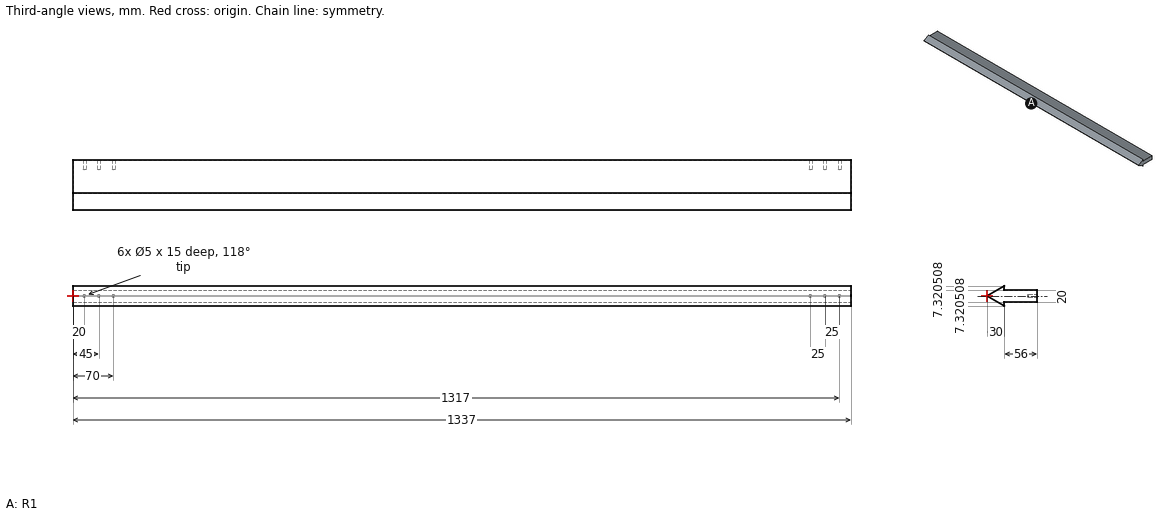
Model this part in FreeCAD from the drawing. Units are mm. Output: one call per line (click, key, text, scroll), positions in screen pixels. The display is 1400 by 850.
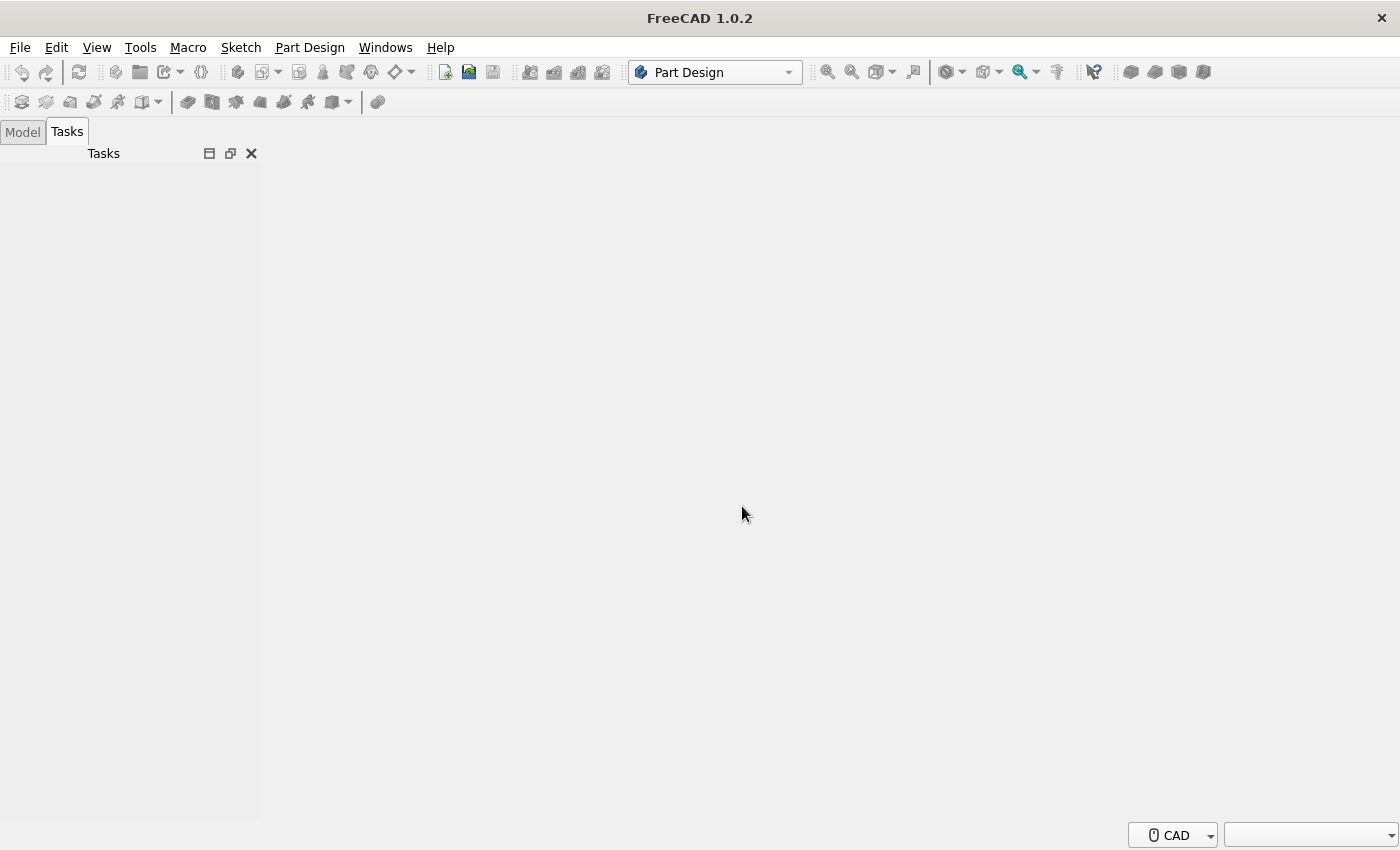
click(446, 72)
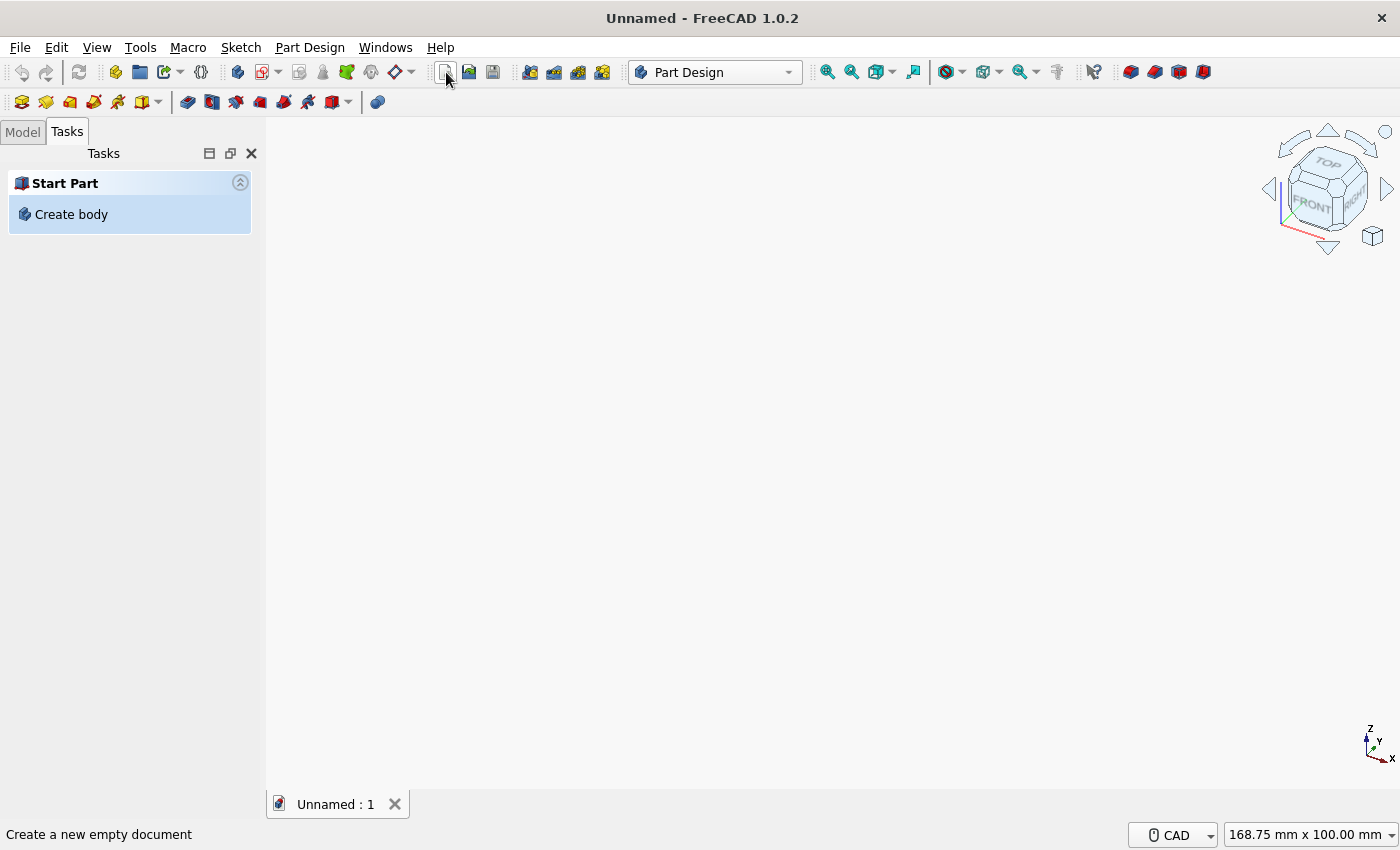
click(262, 72)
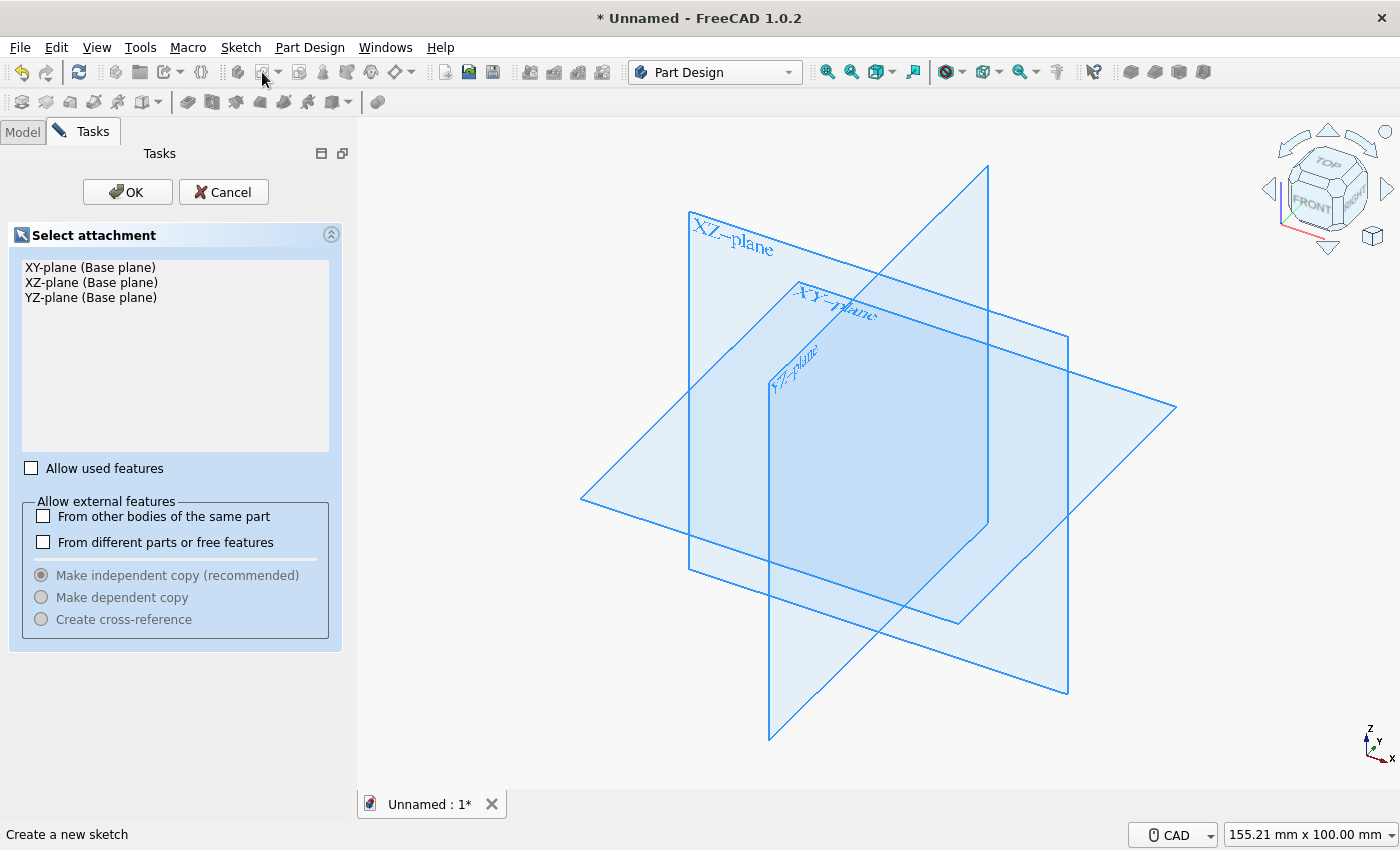
click(82, 298)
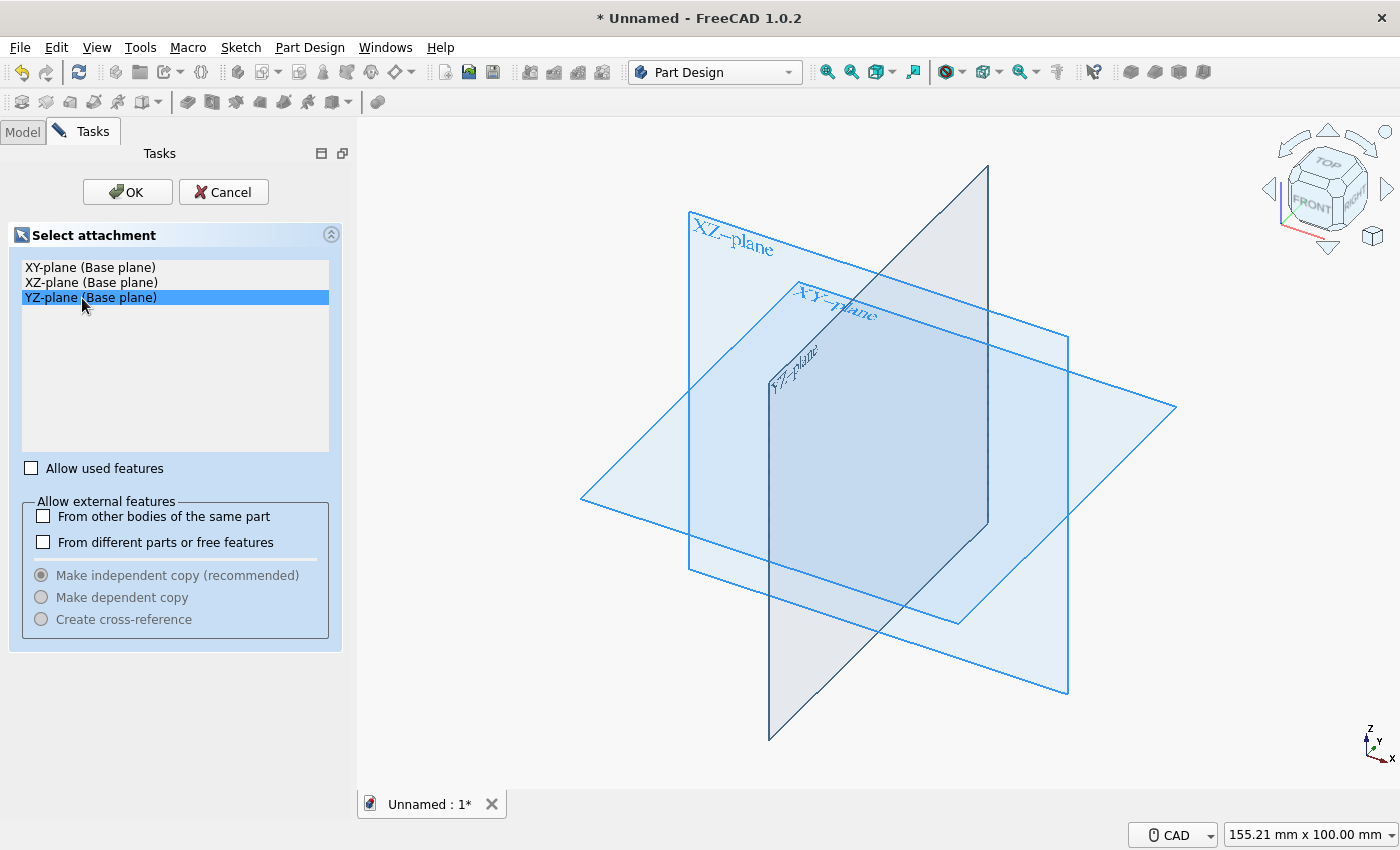
click(128, 192)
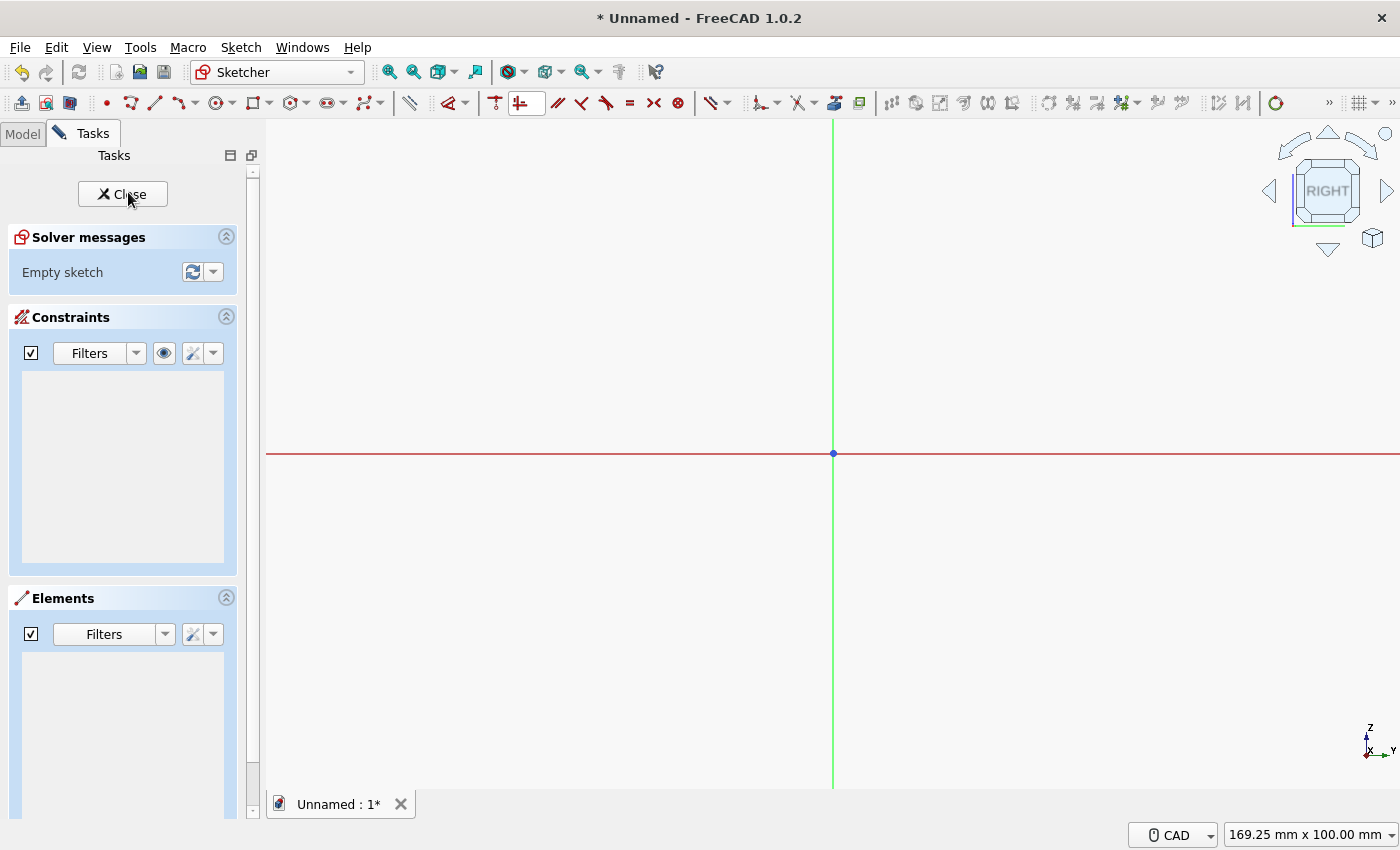
scroll(294, 454, down, 1)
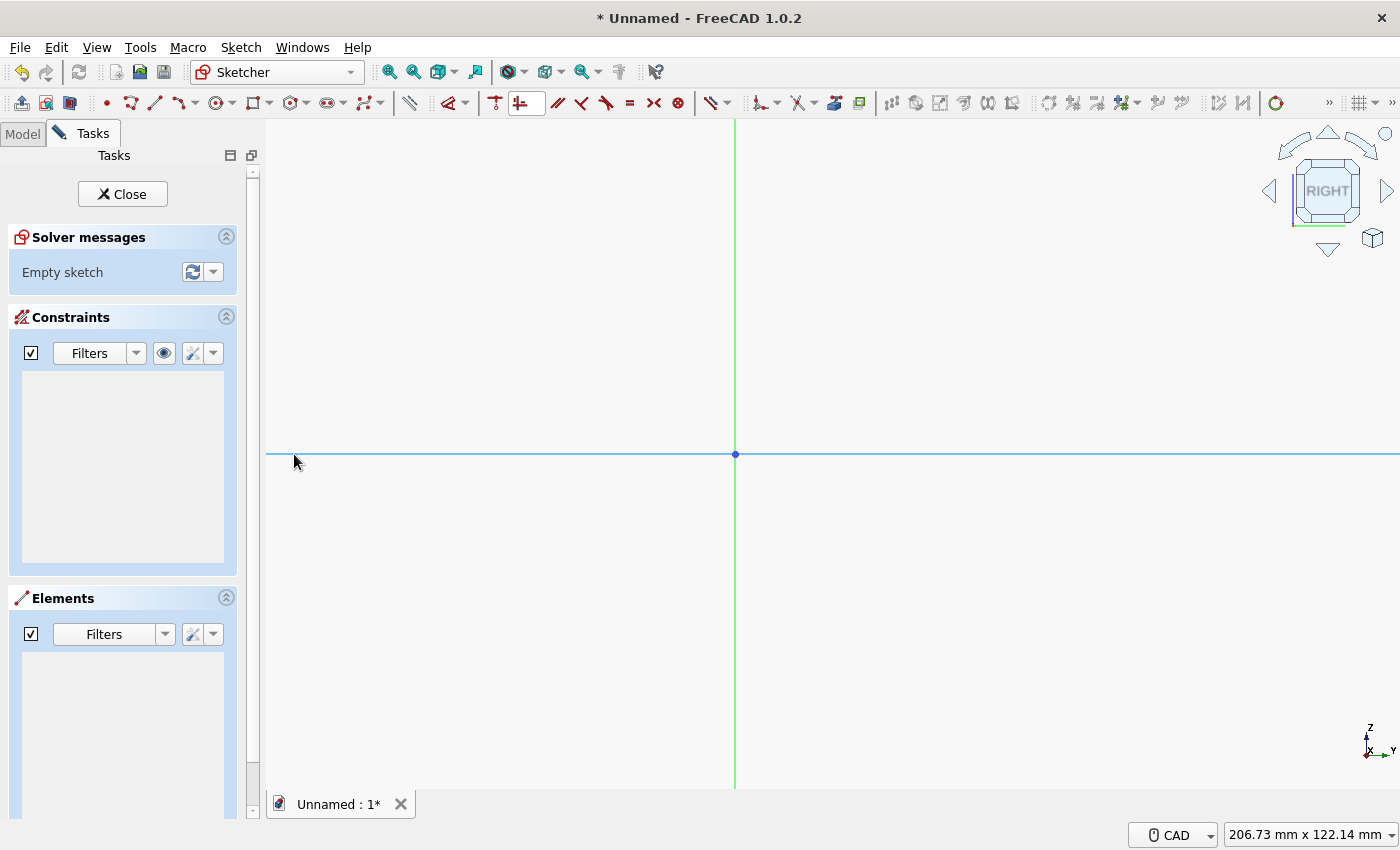
scroll(1235, 454, up, 2)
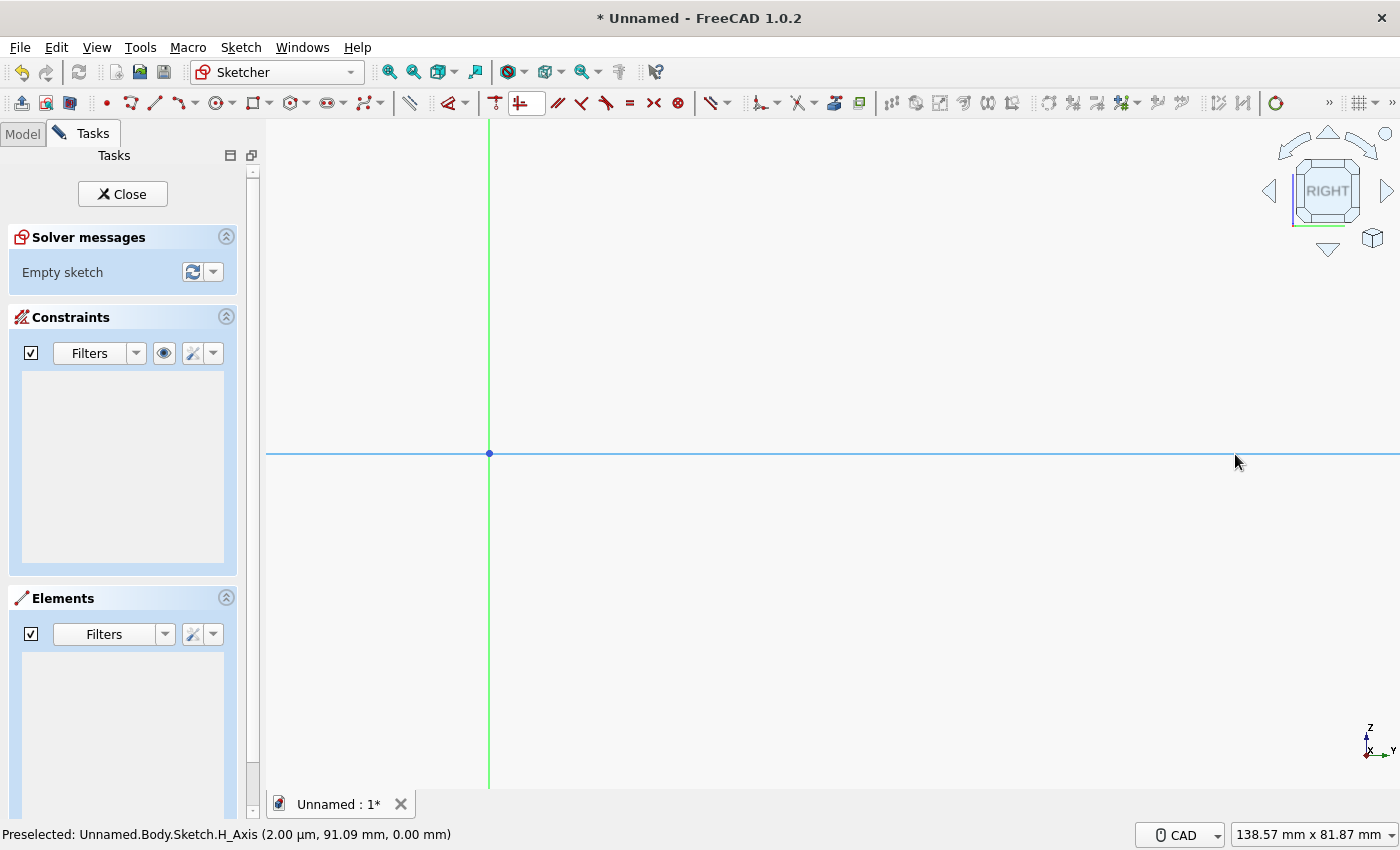
click(132, 104)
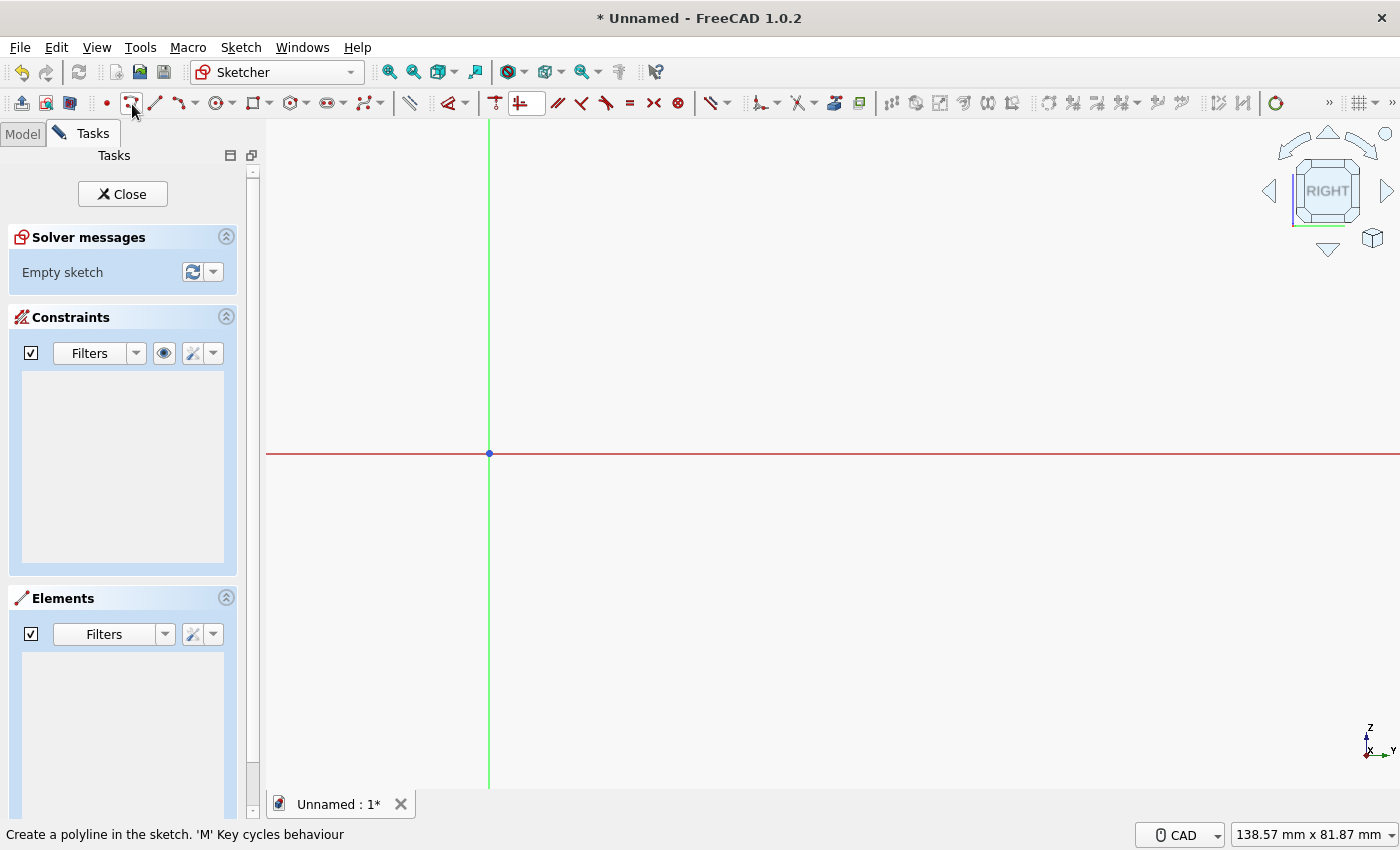
click(489, 454)
click(735, 596)
click(735, 536)
click(1193, 536)
click(1193, 372)
click(735, 372)
click(735, 312)
click(489, 454)
key(Escape)
key(Escape)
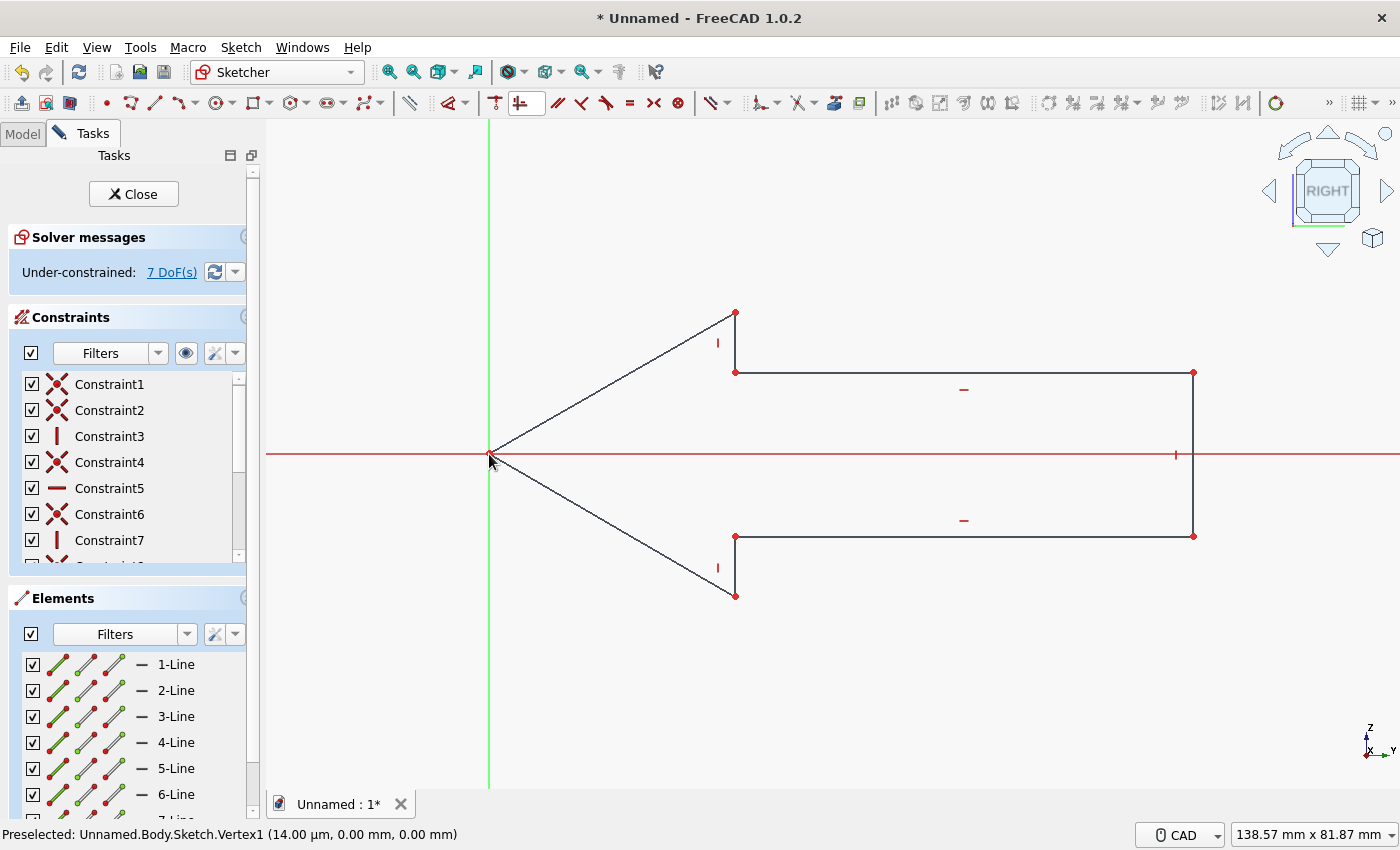
click(735, 537)